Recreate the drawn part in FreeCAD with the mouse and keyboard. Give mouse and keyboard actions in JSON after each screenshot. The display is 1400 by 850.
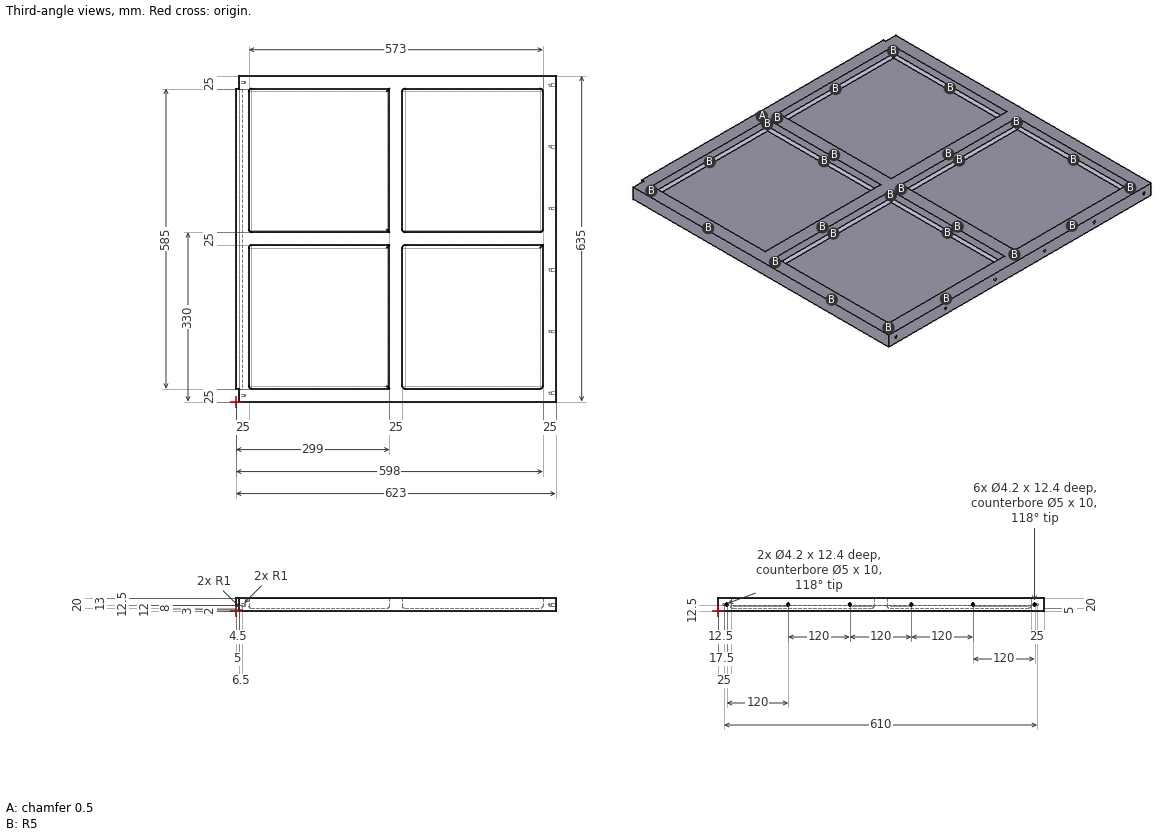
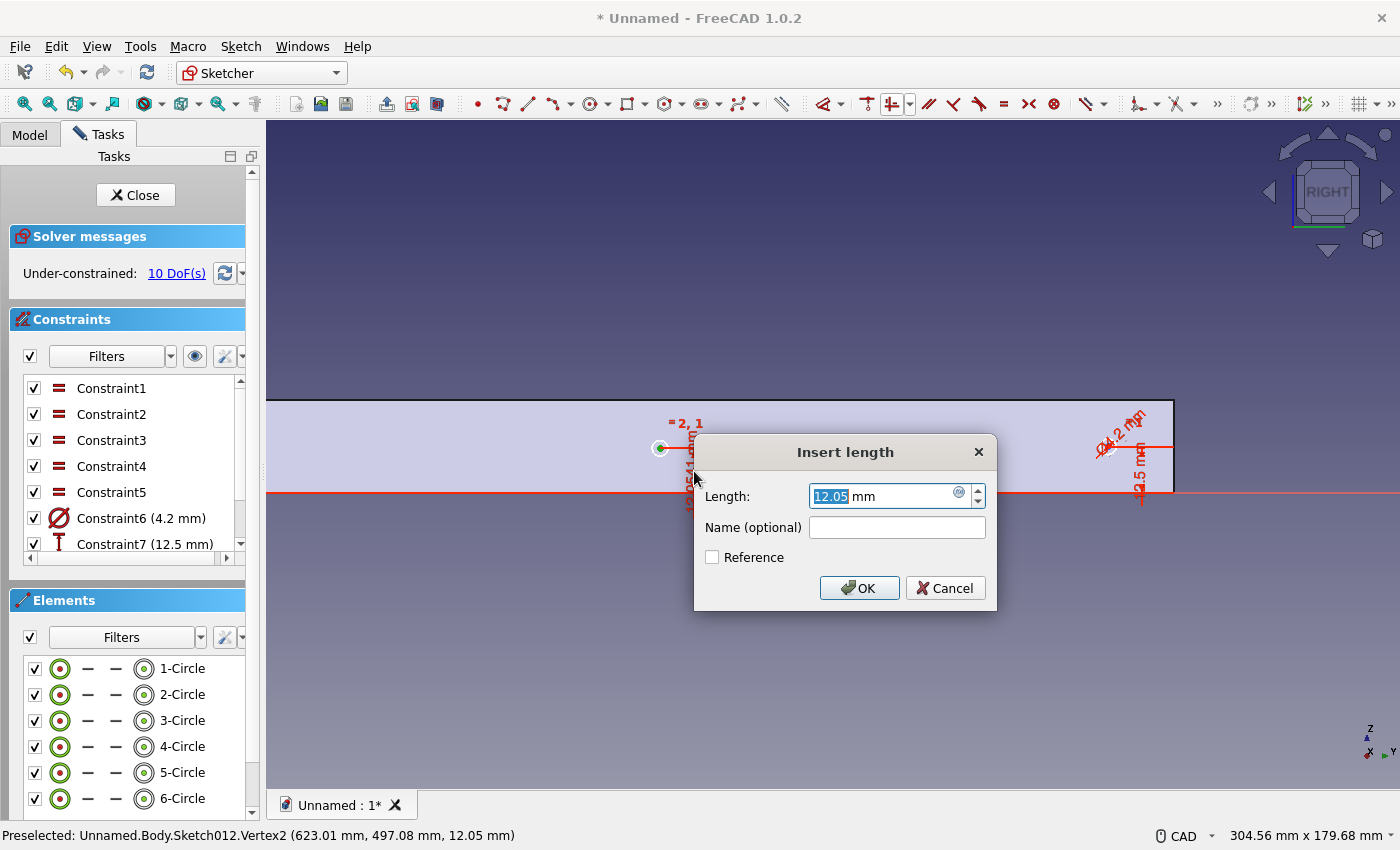
{"action": "type", "text": "12.5"}
{"action": "key", "text": "Return"}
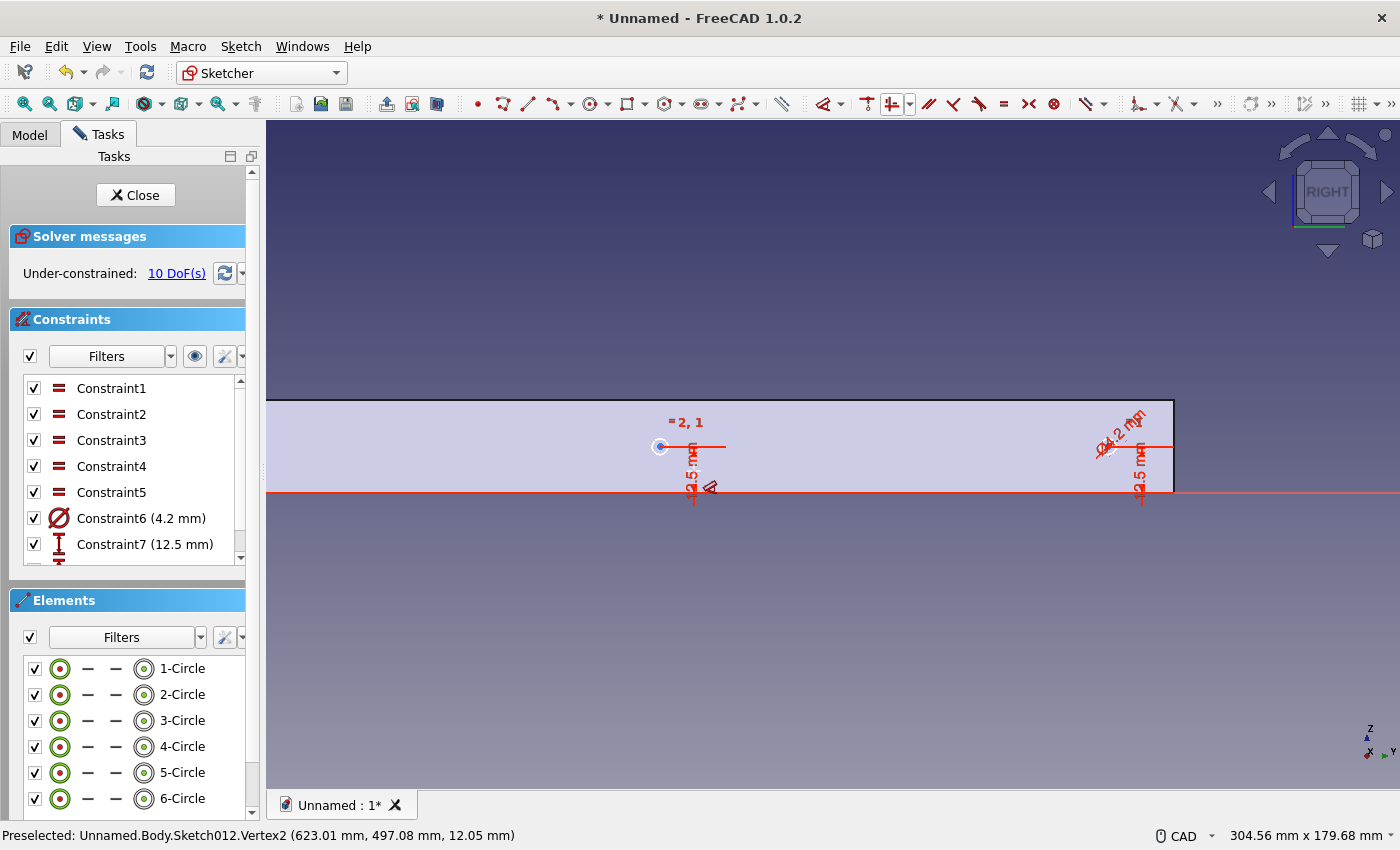
{"action": "scroll", "coordinate": [1110, 449], "scroll_direction": "down", "scroll_amount": 6}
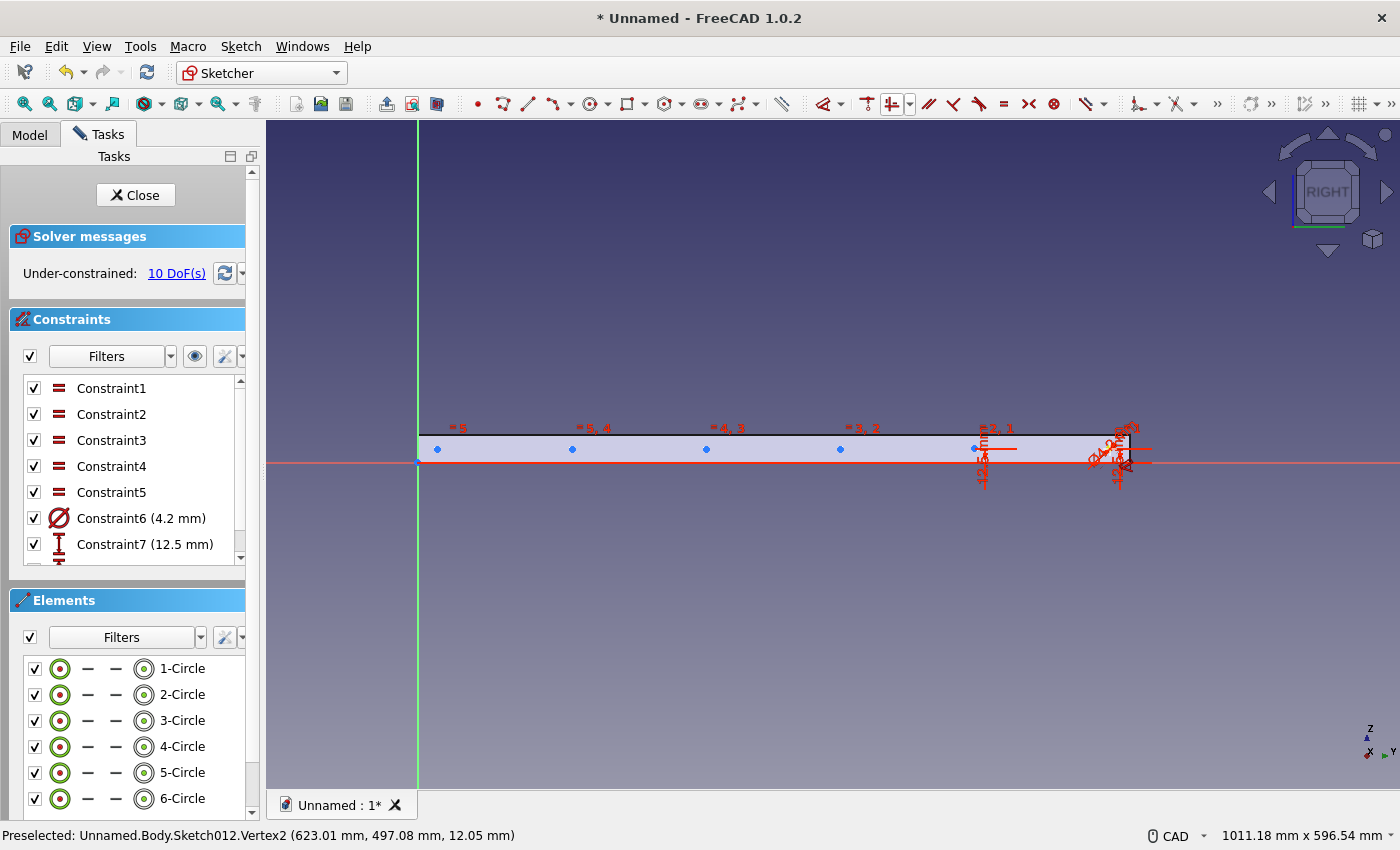
{"action": "scroll", "coordinate": [841, 449], "scroll_direction": "up", "scroll_amount": 6}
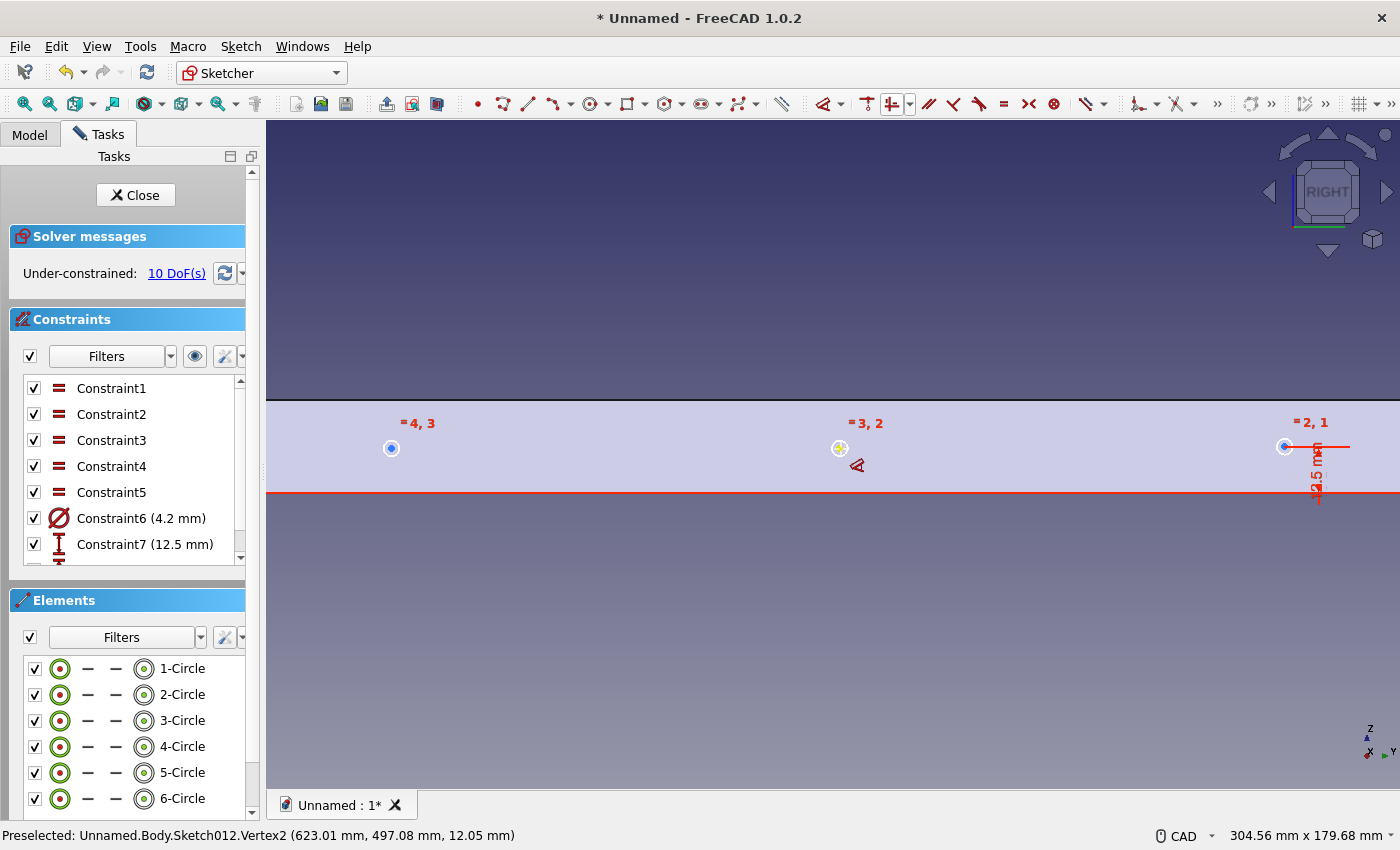
{"action": "left_click", "coordinate": [840, 448]}
{"action": "left_click", "coordinate": [874, 471]}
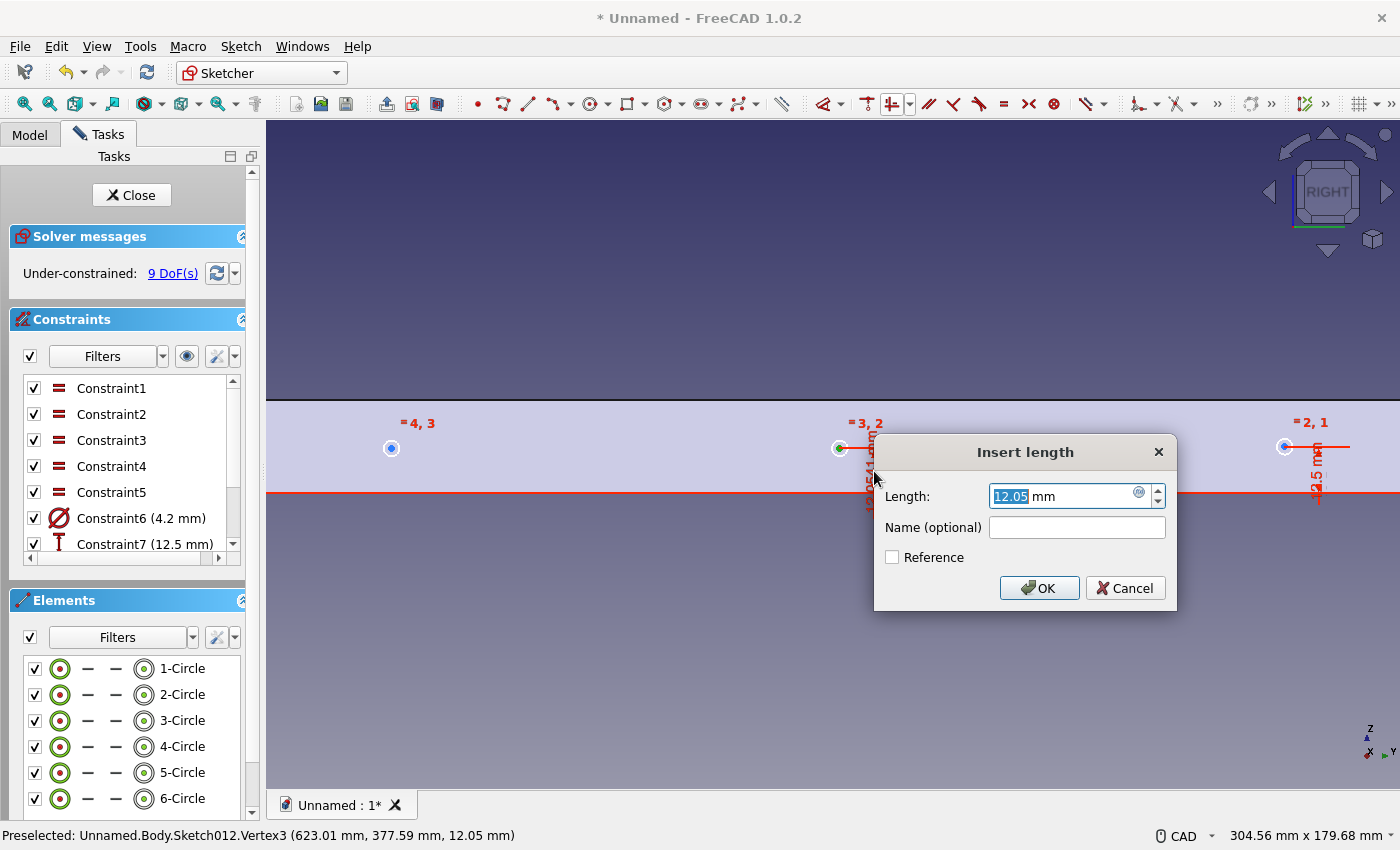
{"action": "type", "text": "12.5"}
{"action": "key", "text": "Return"}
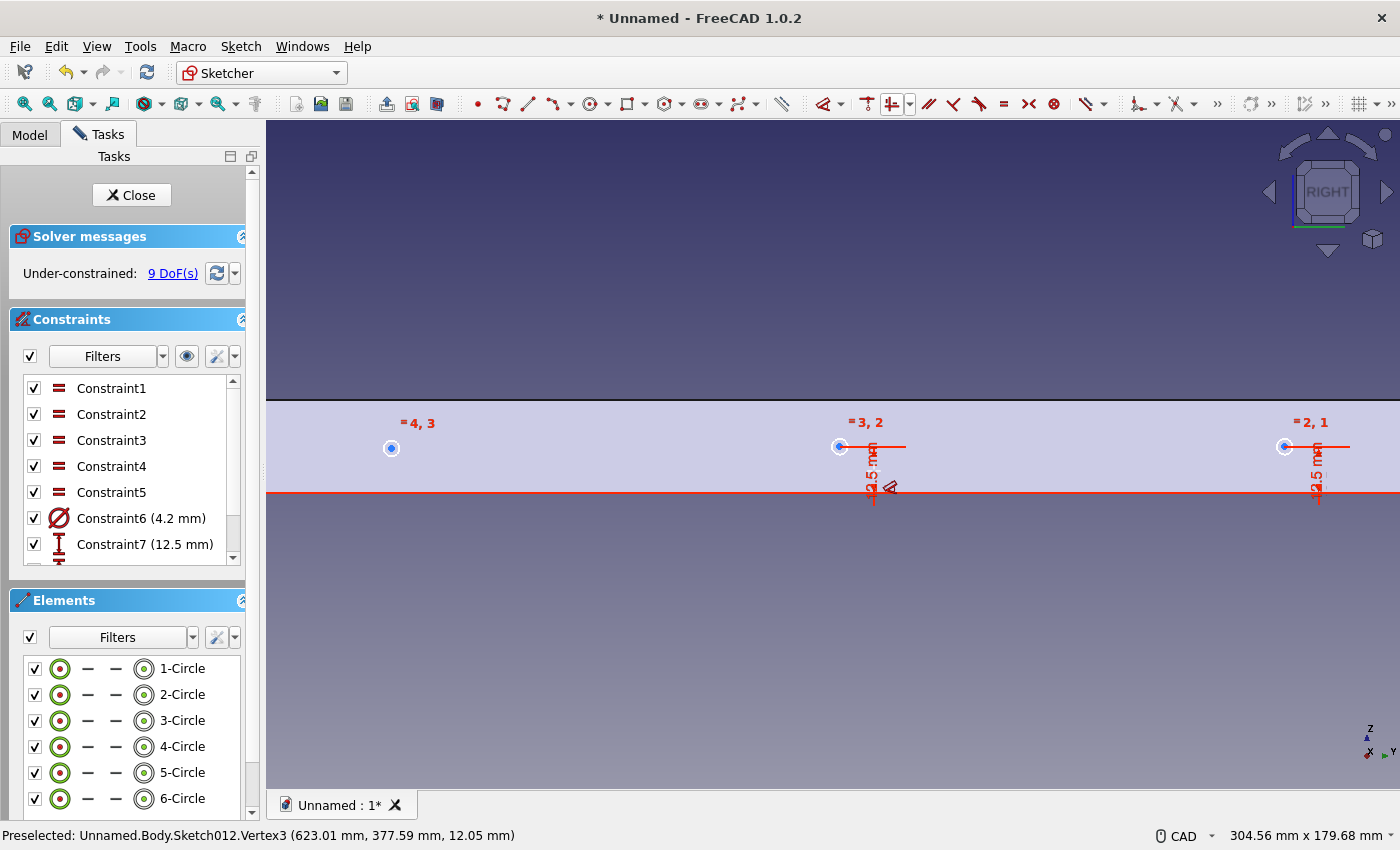
{"action": "left_click", "coordinate": [392, 448]}
{"action": "left_click", "coordinate": [426, 471]}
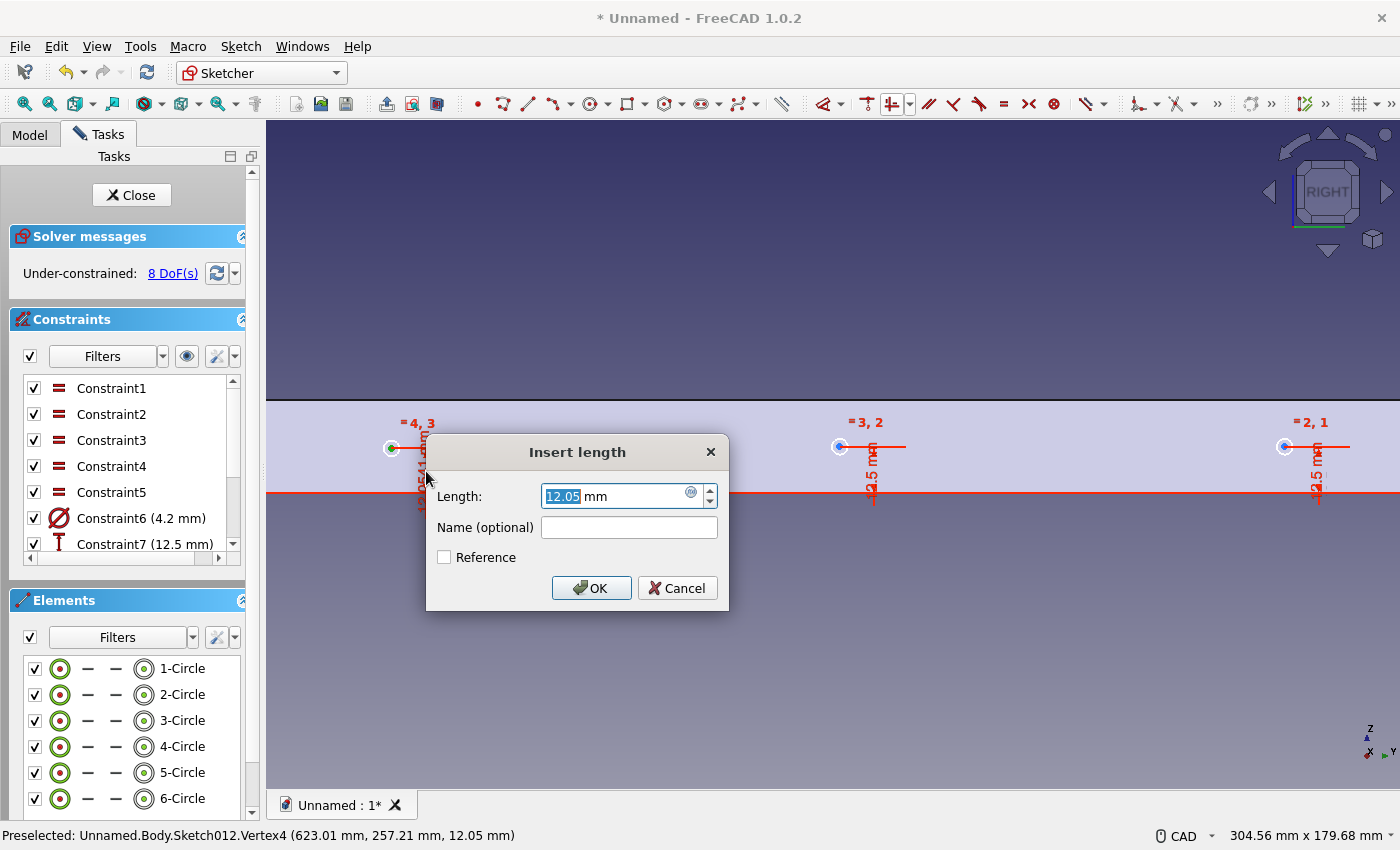
{"action": "type", "text": "12.5"}
{"action": "key", "text": "Return"}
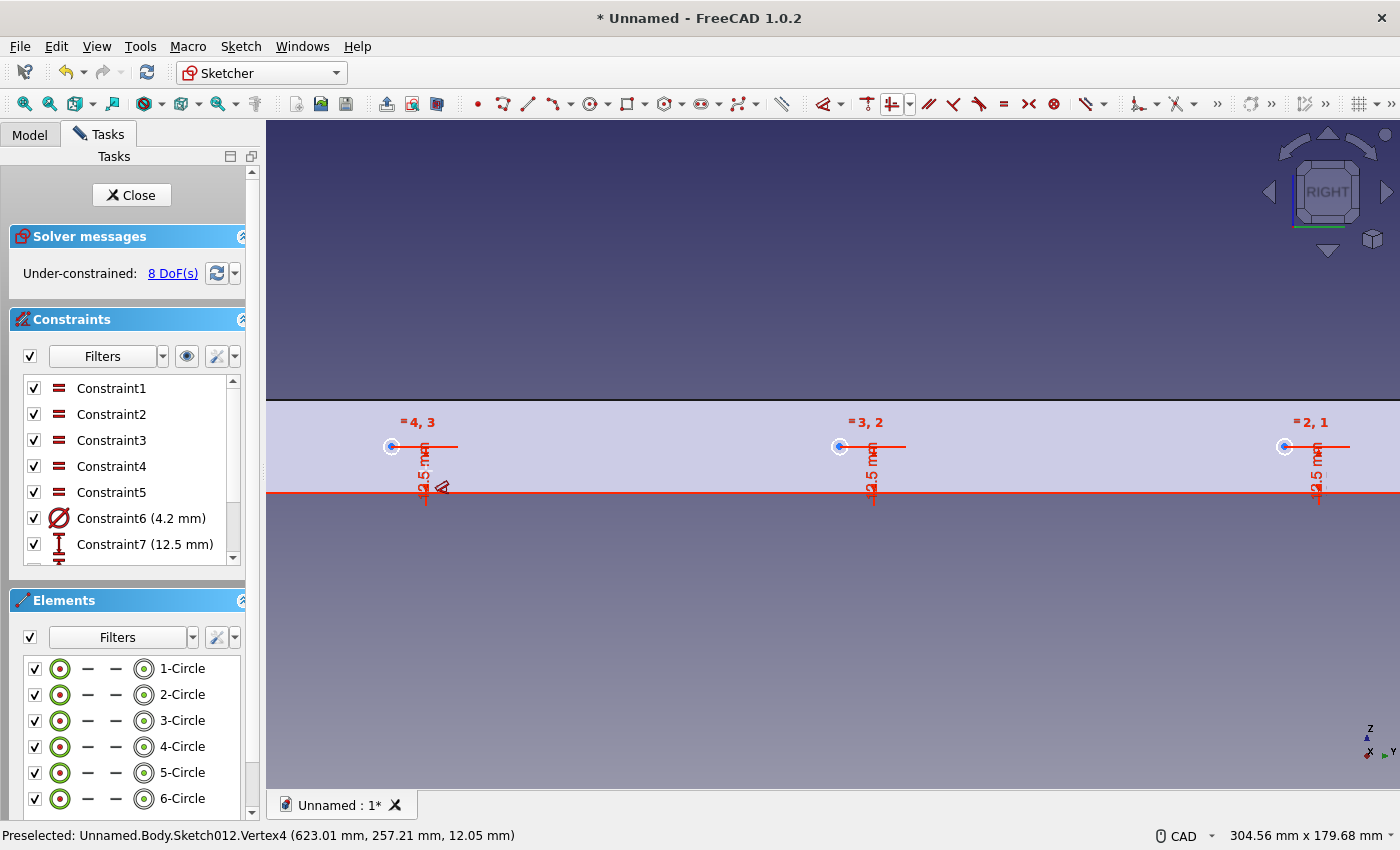
{"action": "scroll", "coordinate": [841, 449], "scroll_direction": "down", "scroll_amount": 6}